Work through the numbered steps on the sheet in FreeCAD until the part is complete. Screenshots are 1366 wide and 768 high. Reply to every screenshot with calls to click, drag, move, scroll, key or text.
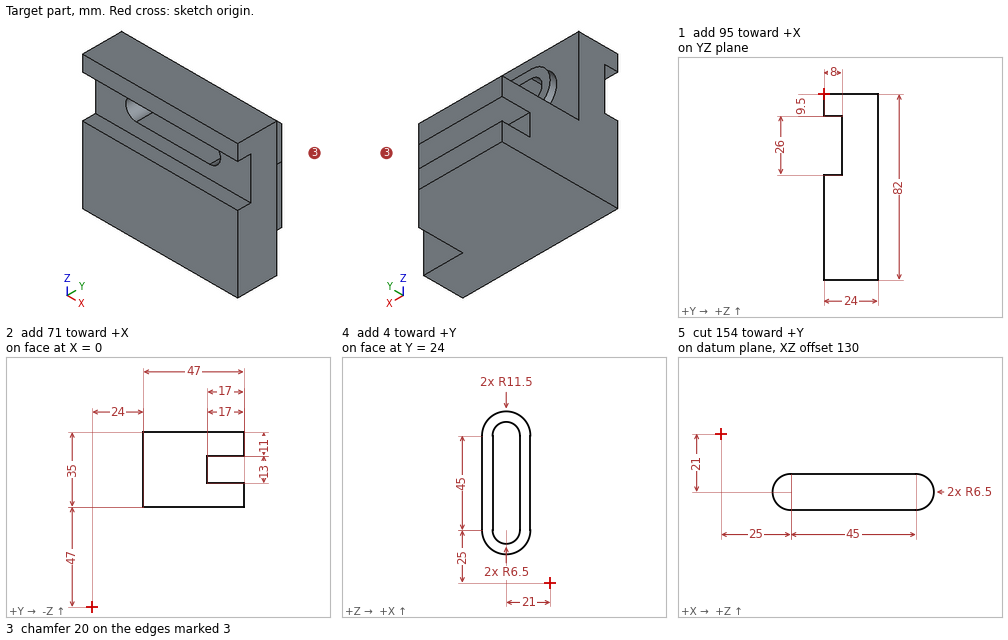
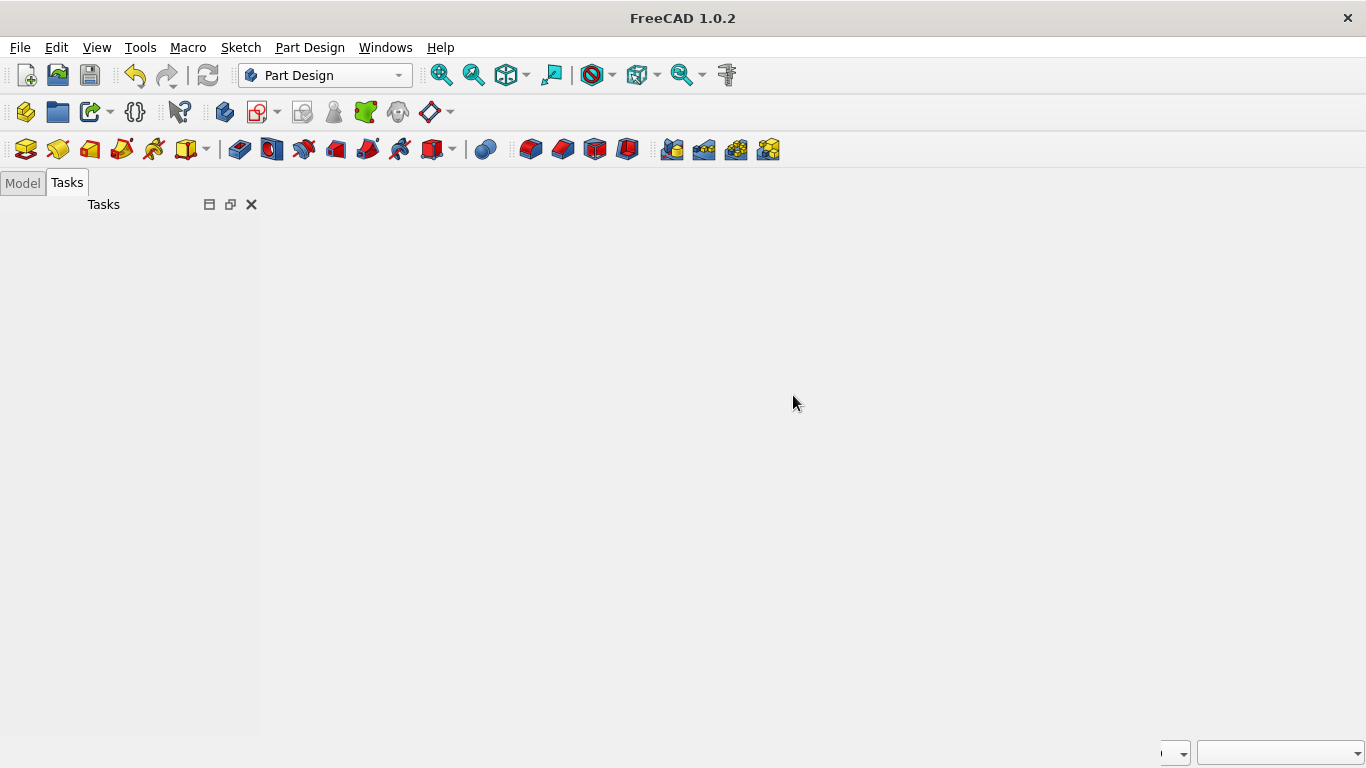
click(26, 76)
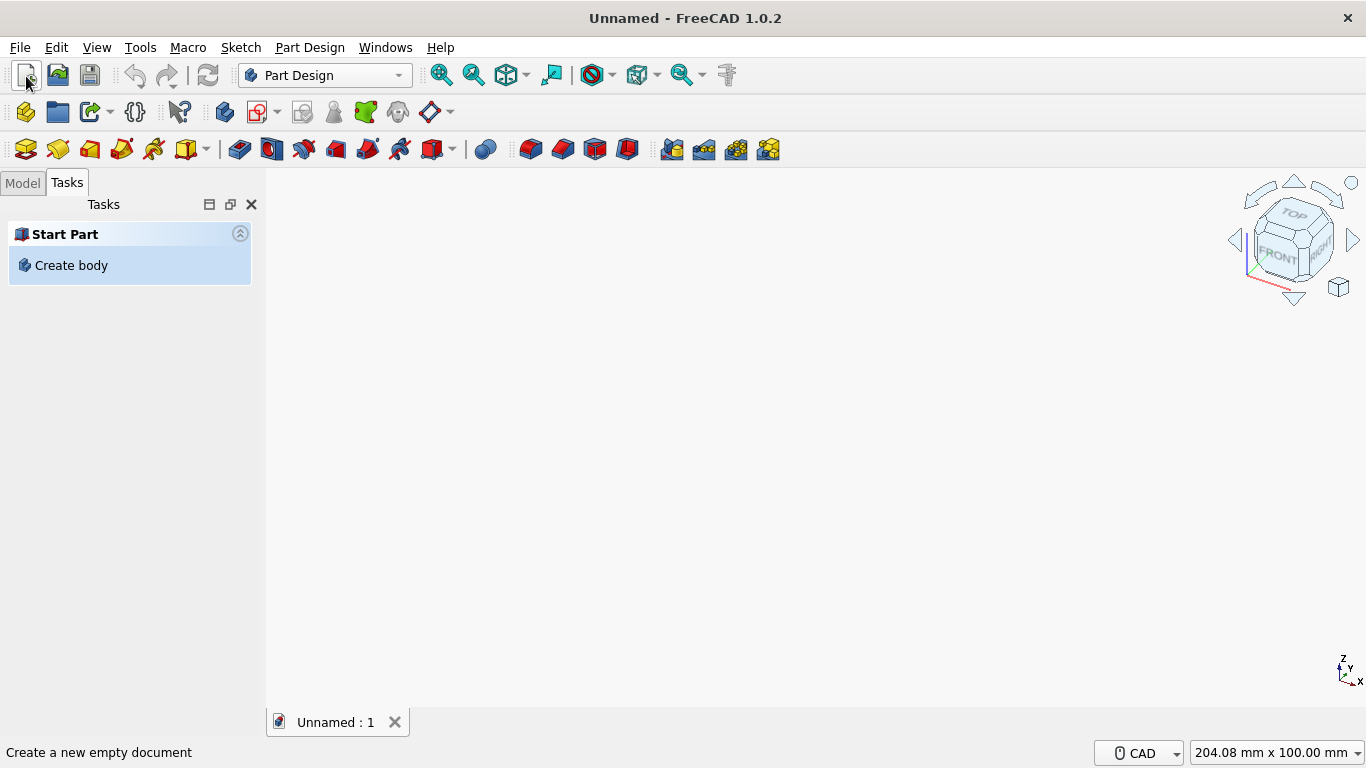
click(258, 112)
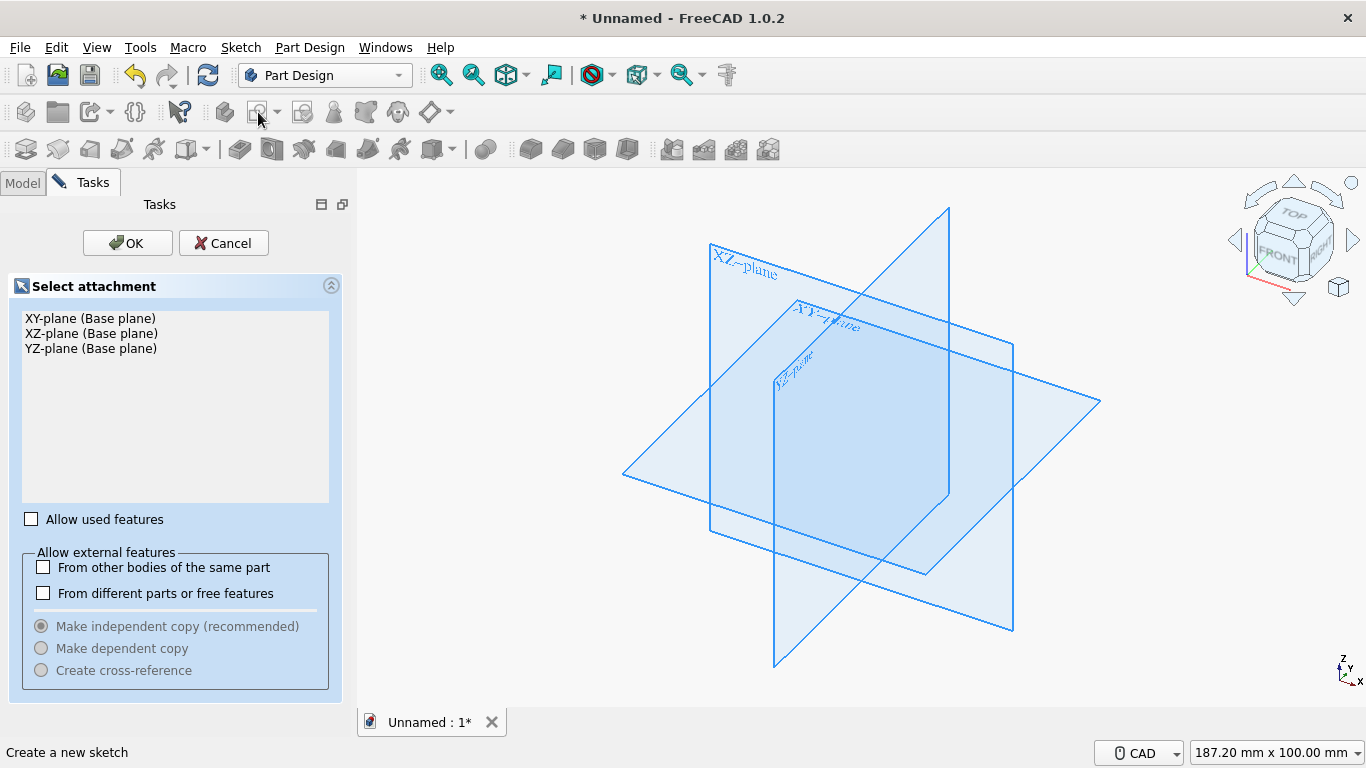
click(82, 348)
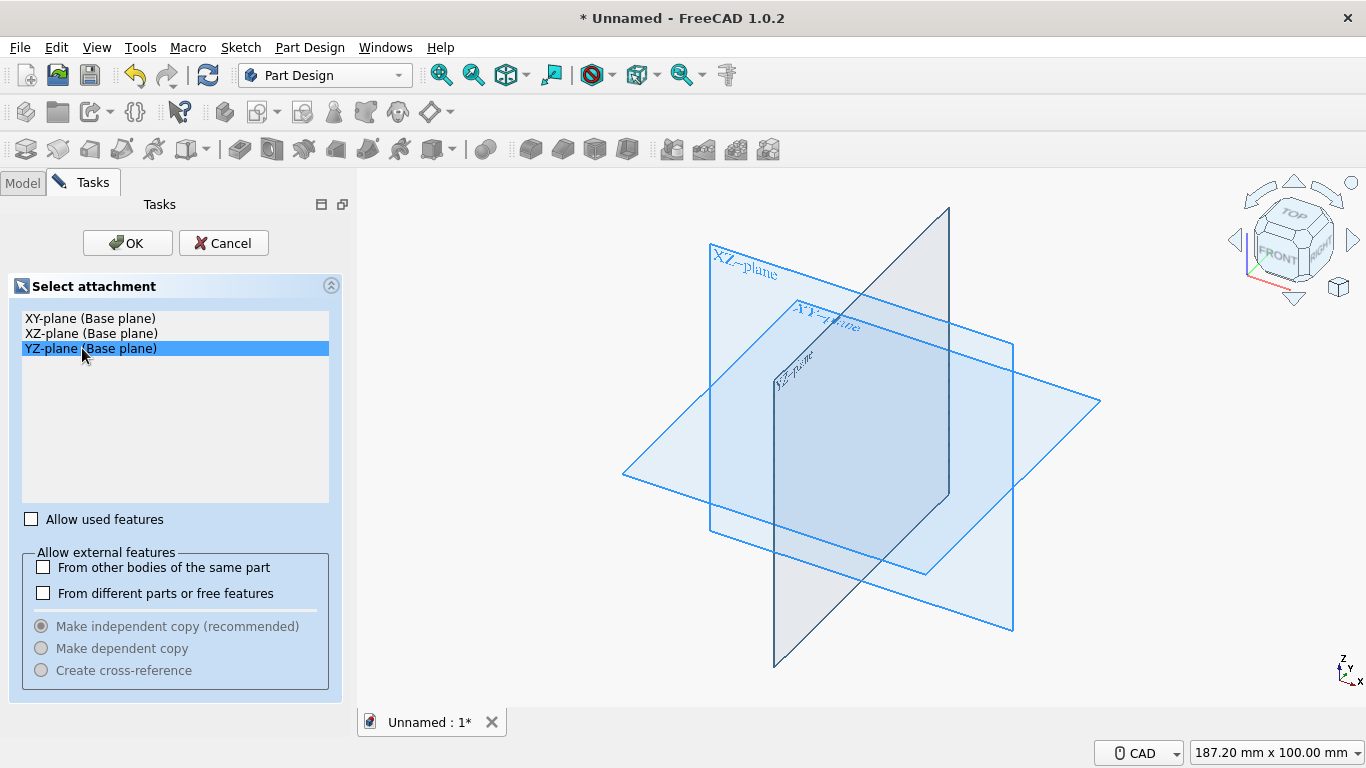
click(128, 243)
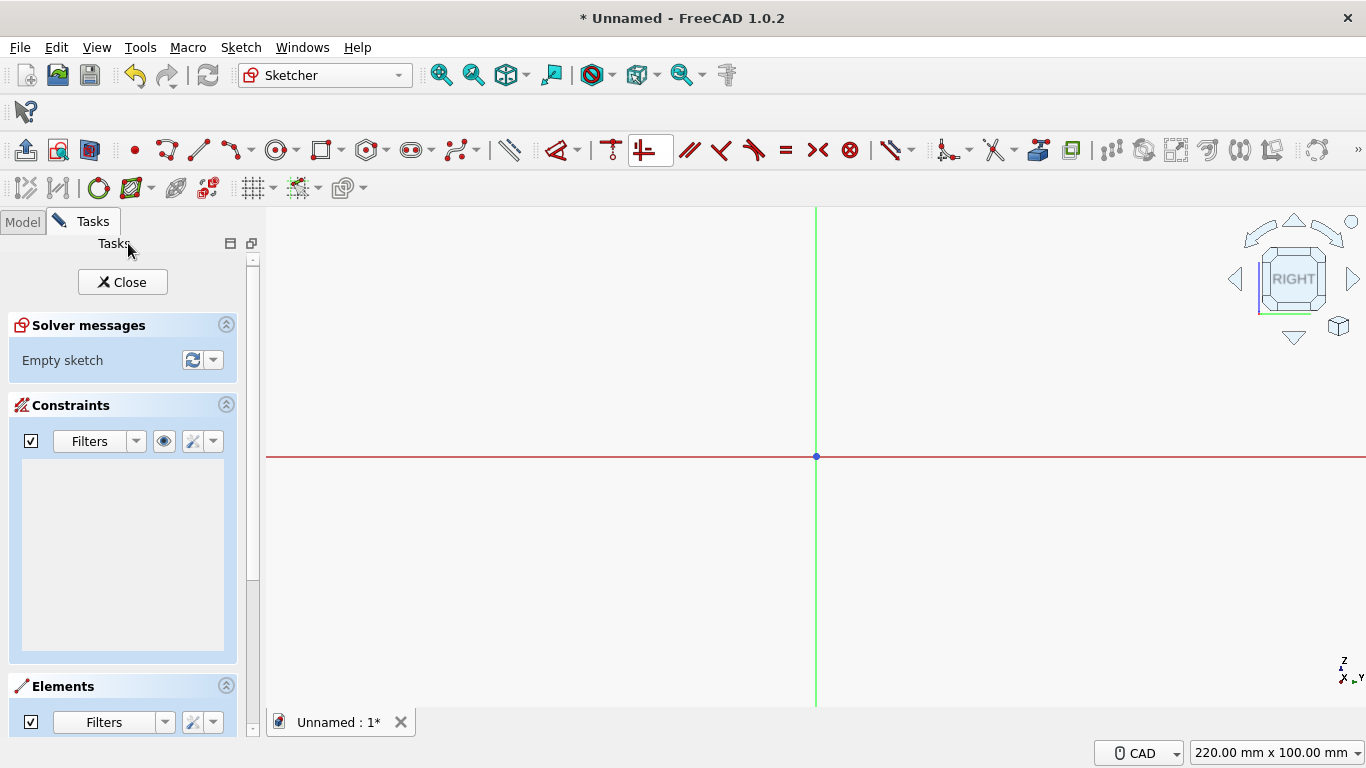
scroll(591, 235, down, 3)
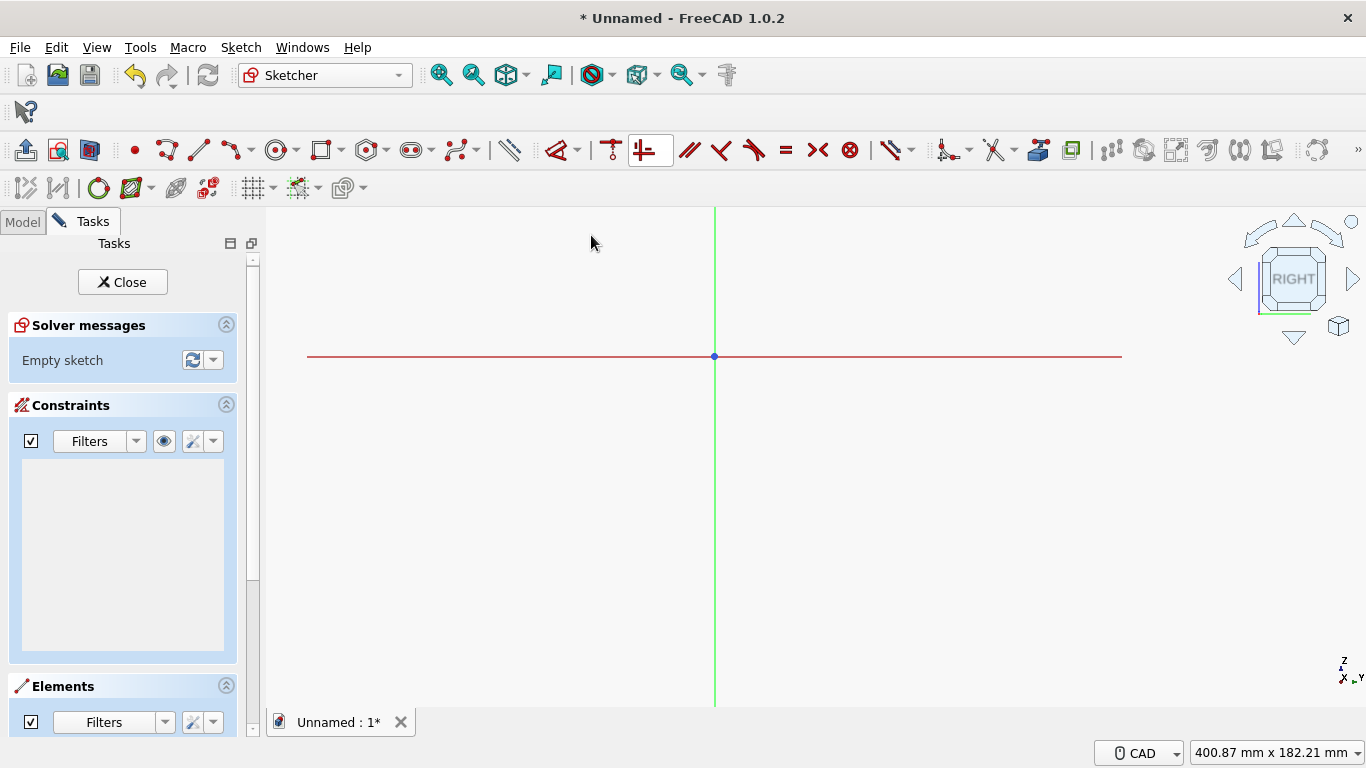
scroll(748, 495, up, 2)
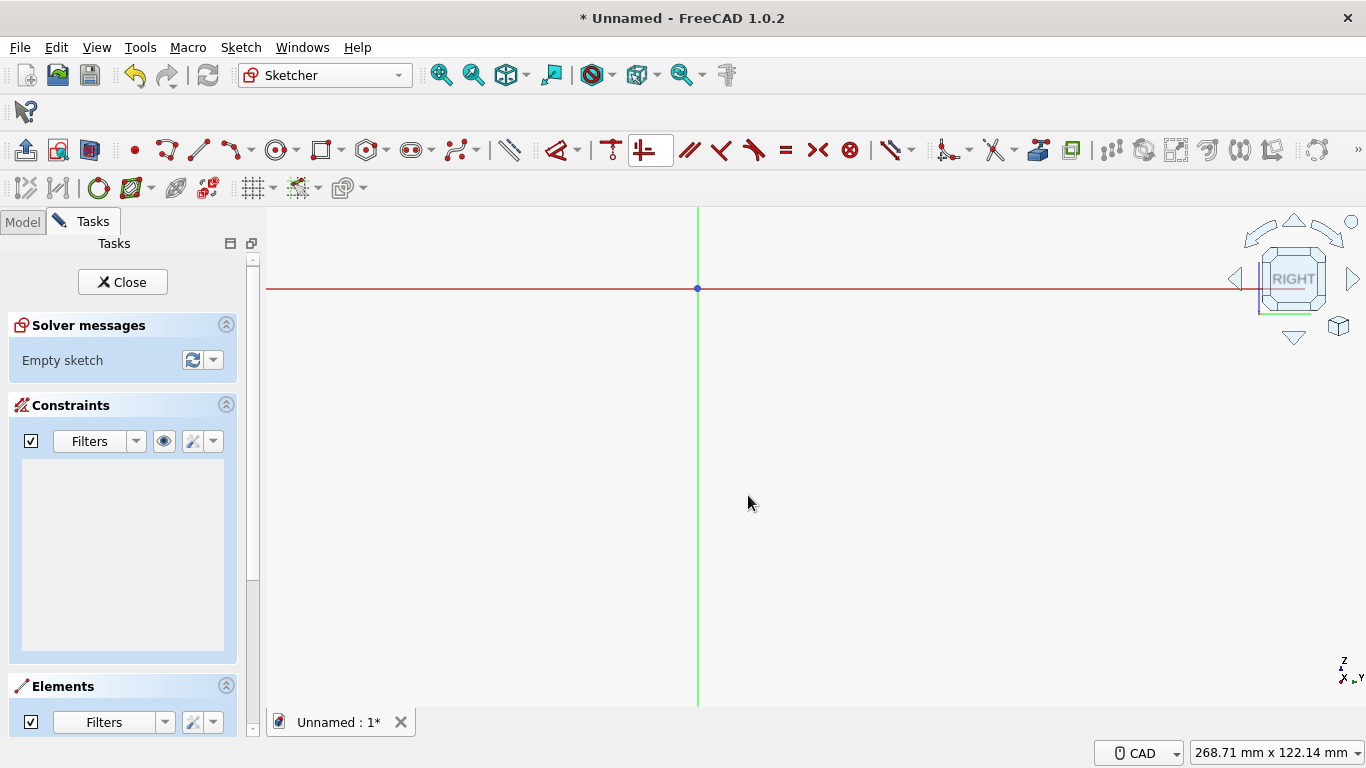
click(168, 150)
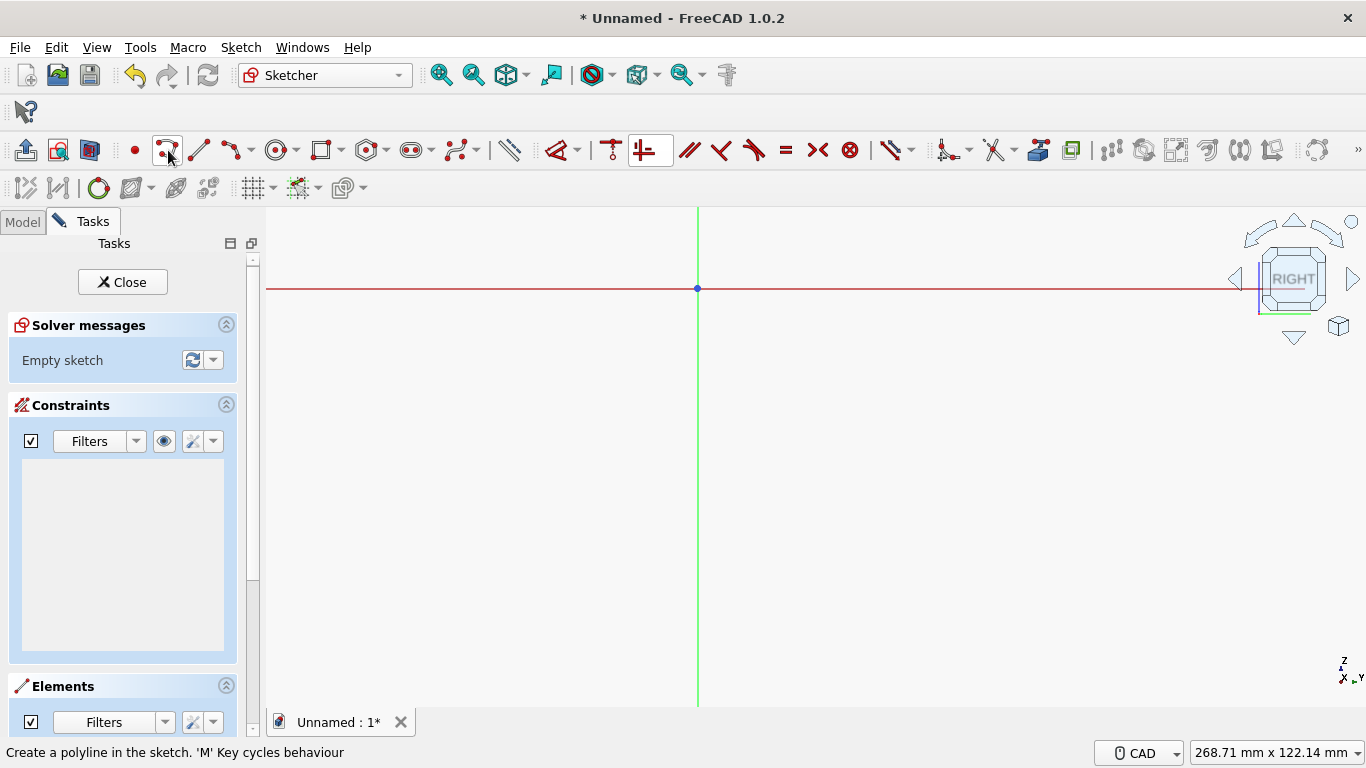
click(698, 289)
click(707, 328)
click(731, 328)
click(731, 434)
click(698, 434)
click(707, 624)
click(796, 624)
click(796, 298)
click(698, 289)
key(Escape)
key(Escape)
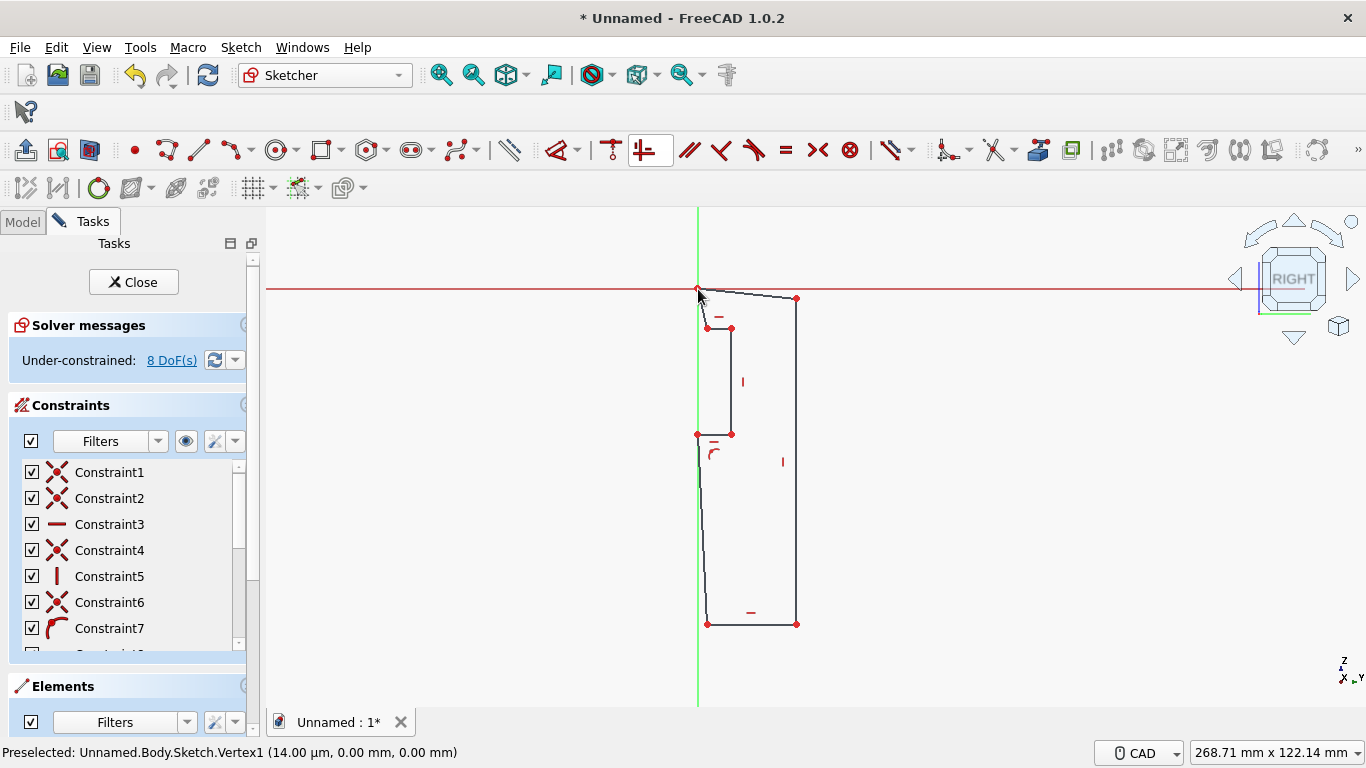
click(701, 301)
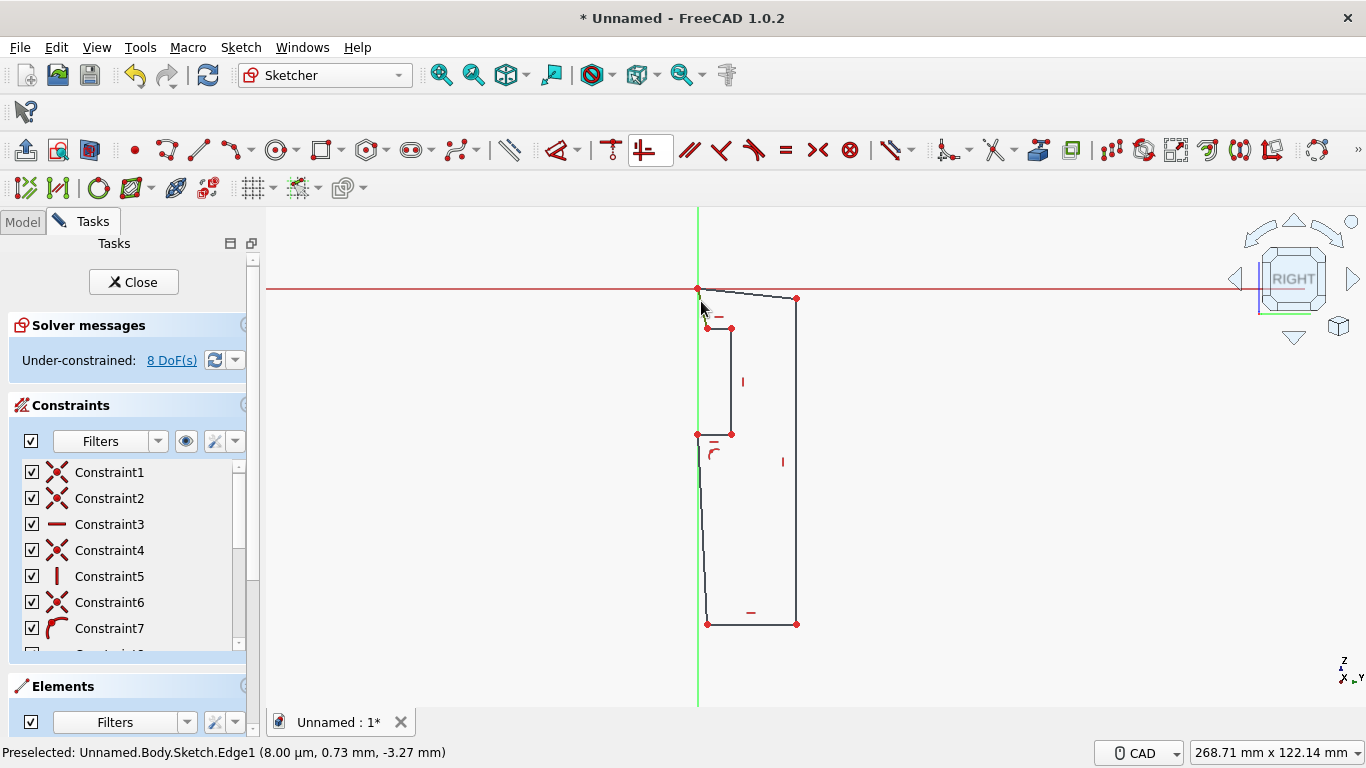
key(v)